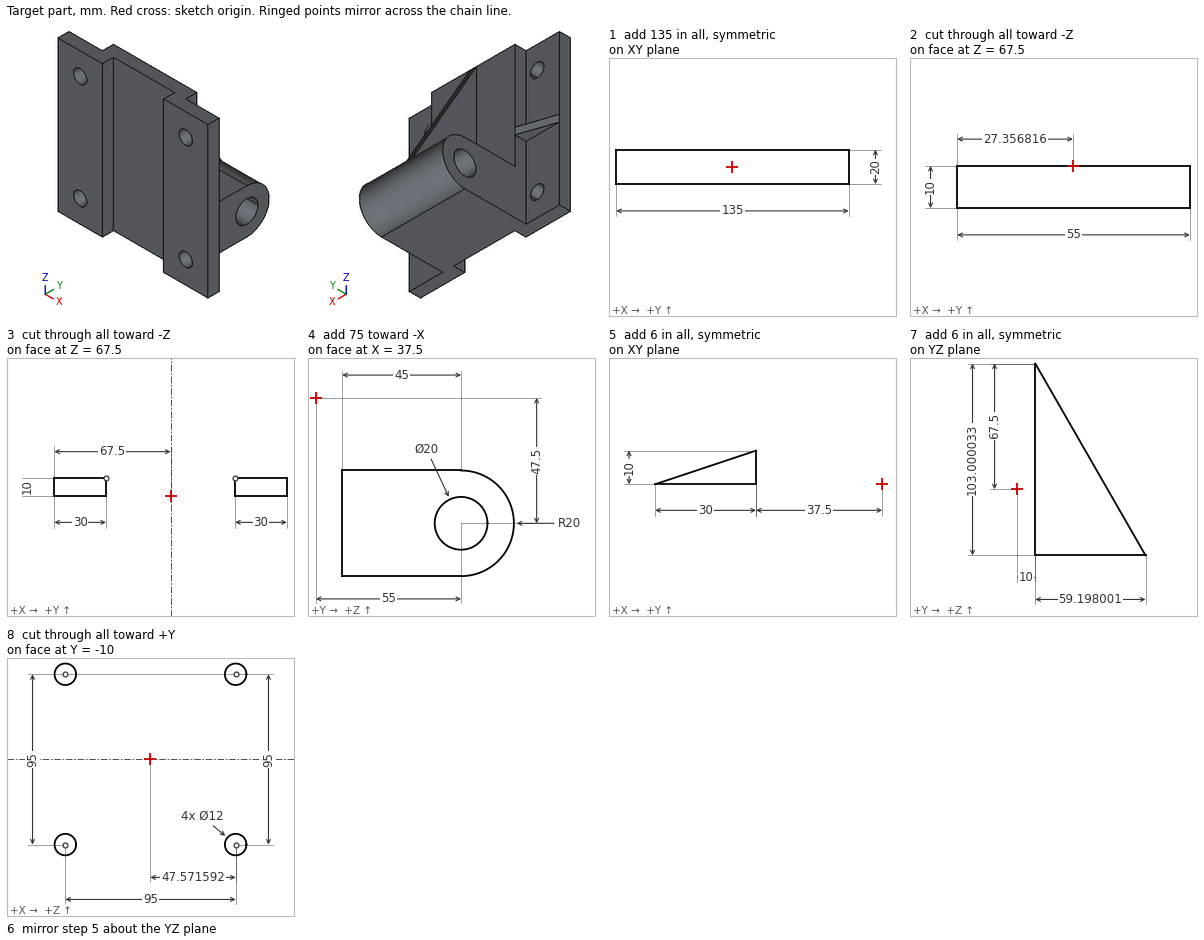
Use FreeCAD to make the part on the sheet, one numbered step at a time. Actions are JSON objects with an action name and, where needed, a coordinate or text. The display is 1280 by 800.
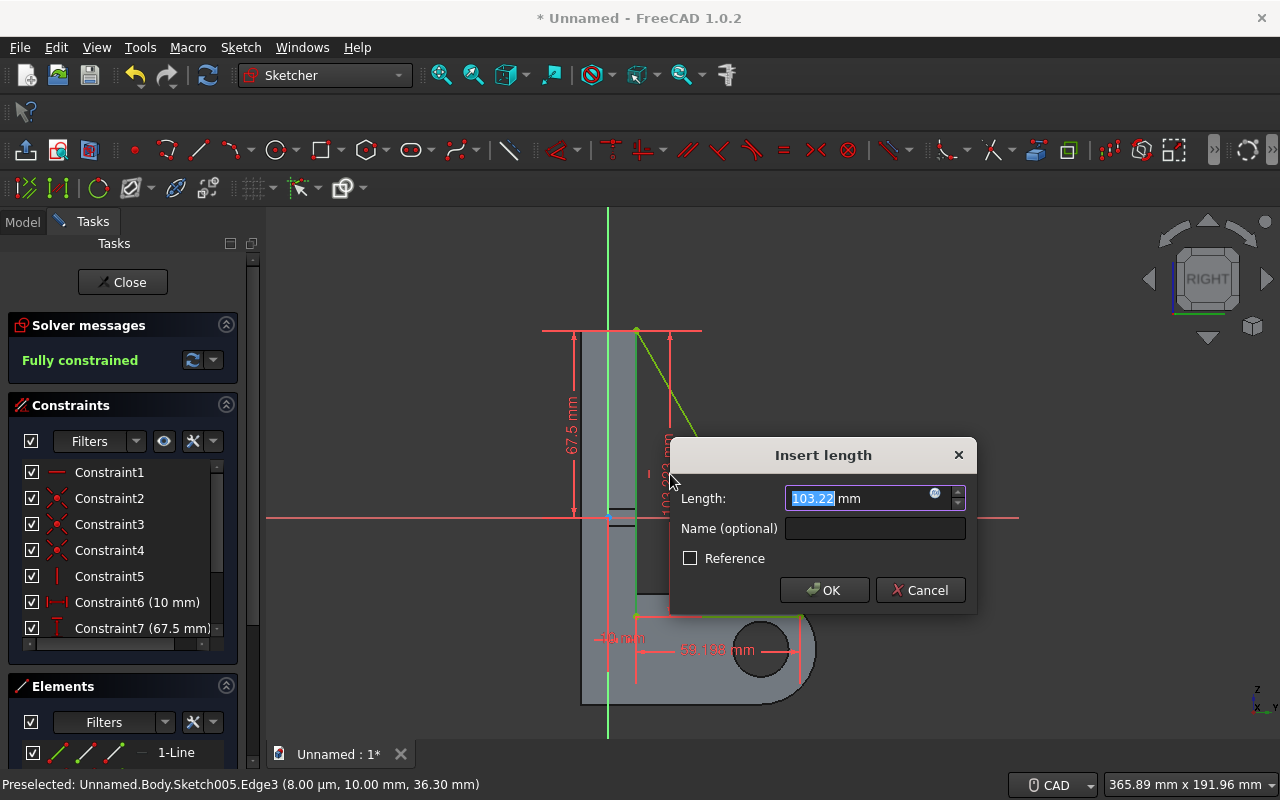
{"action": "type", "text": "103.000033"}
{"action": "key", "text": "Return"}
{"action": "key", "text": "Escape"}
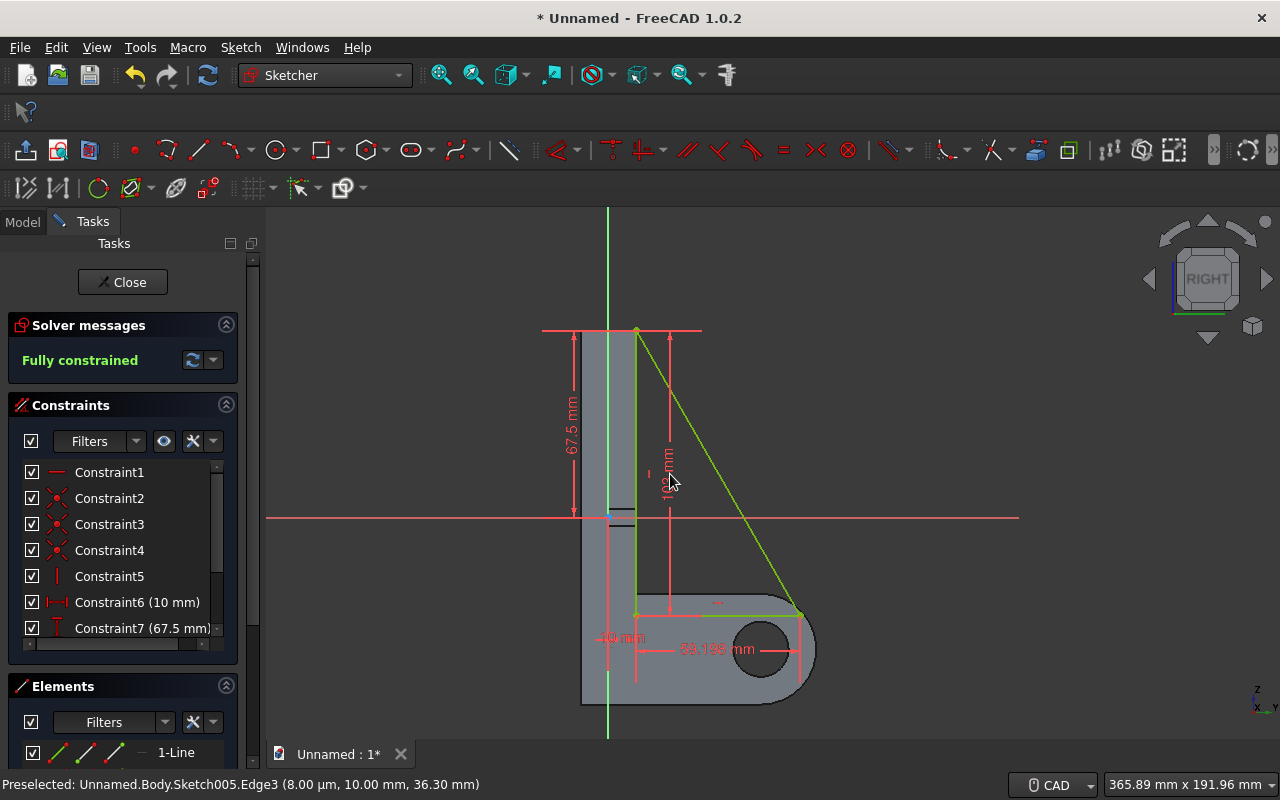
{"action": "left_click", "coordinate": [123, 282]}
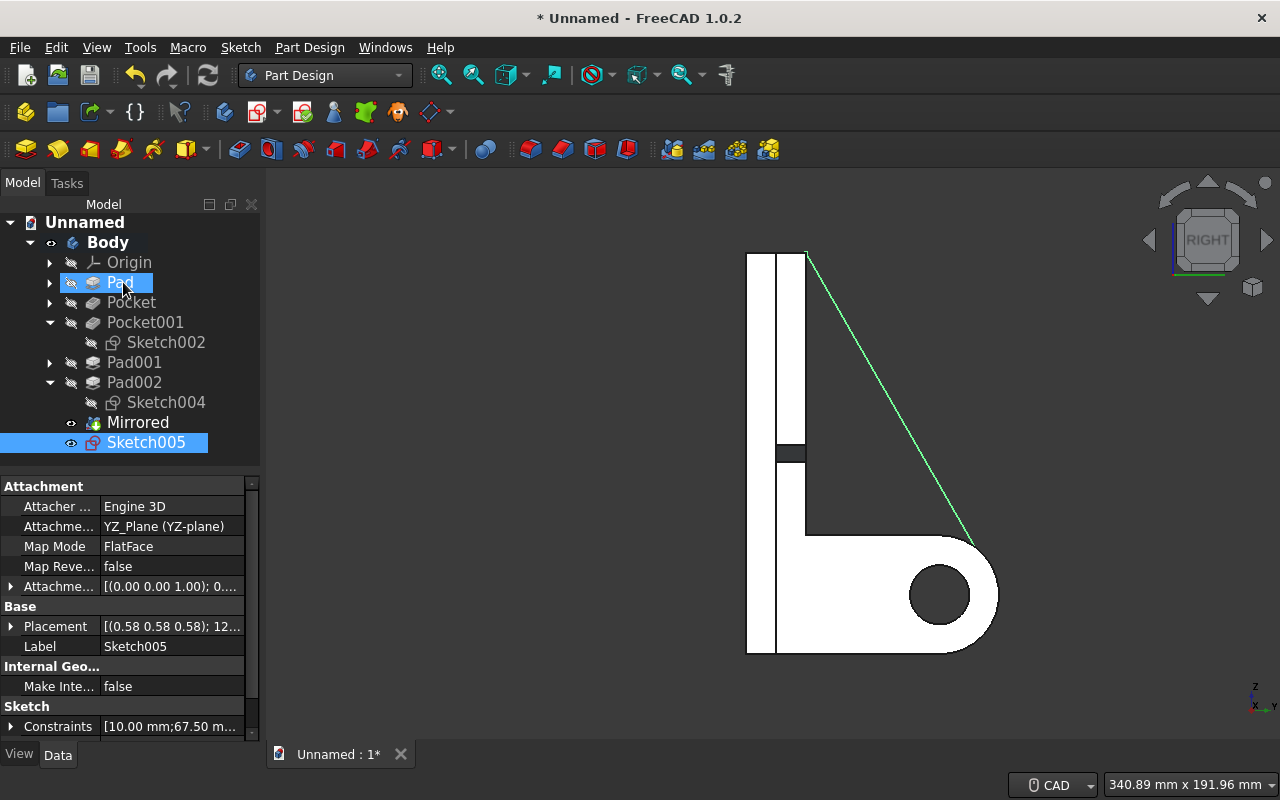
{"action": "left_click", "coordinate": [26, 150]}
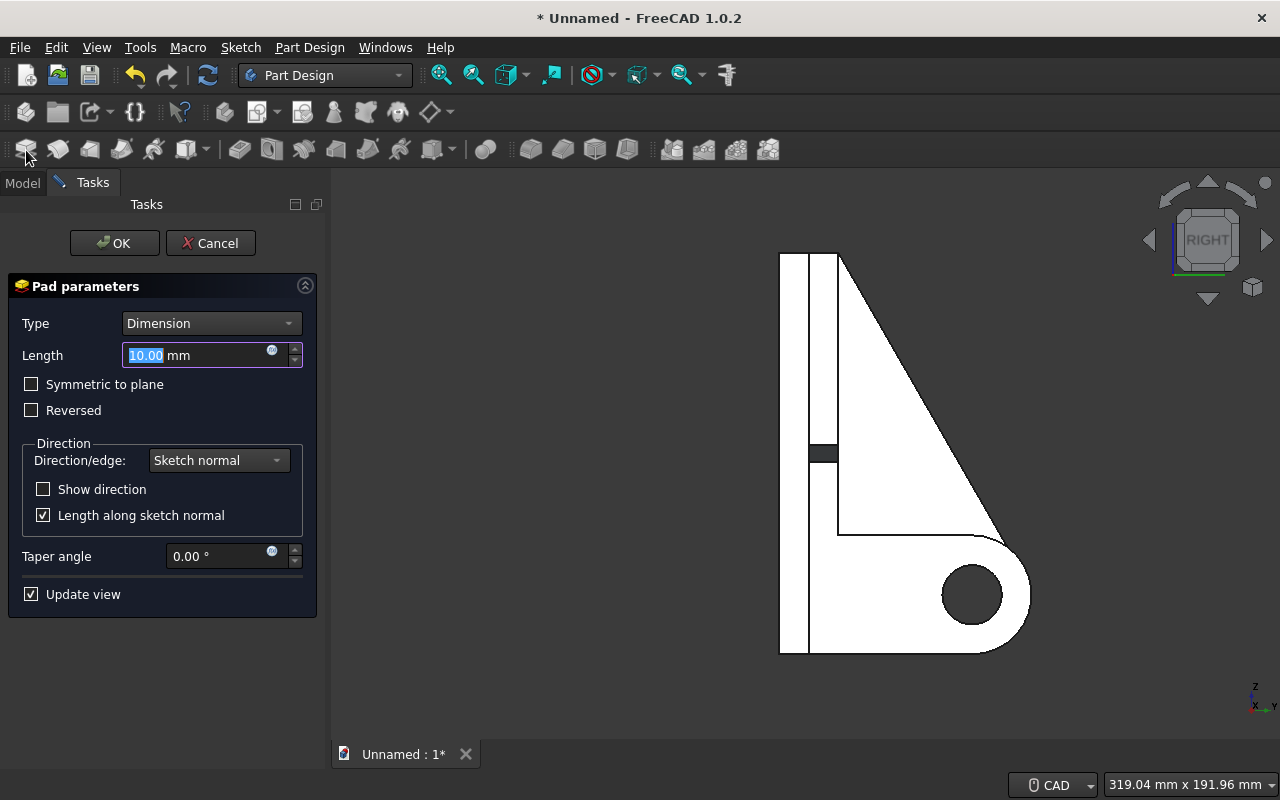
{"action": "type", "text": "6"}
{"action": "key", "text": "Tab"}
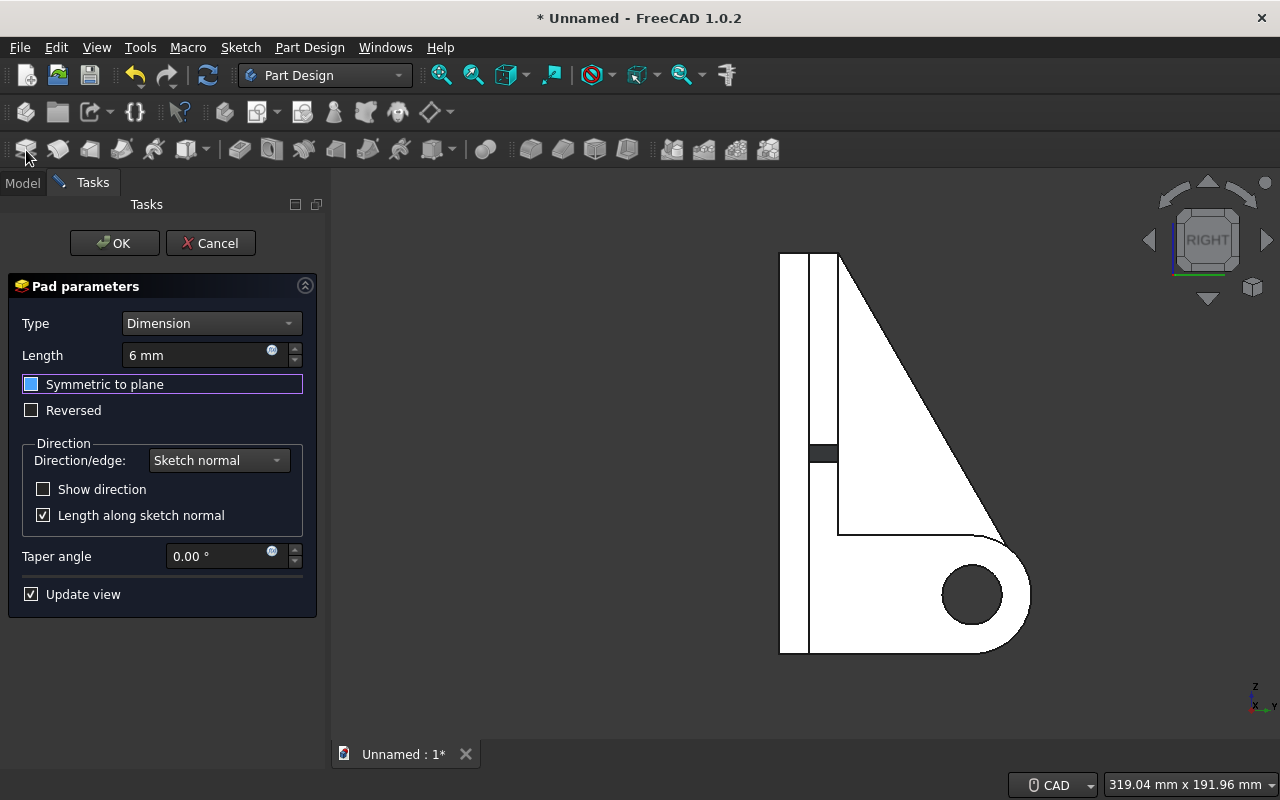
{"action": "left_click", "coordinate": [30, 384]}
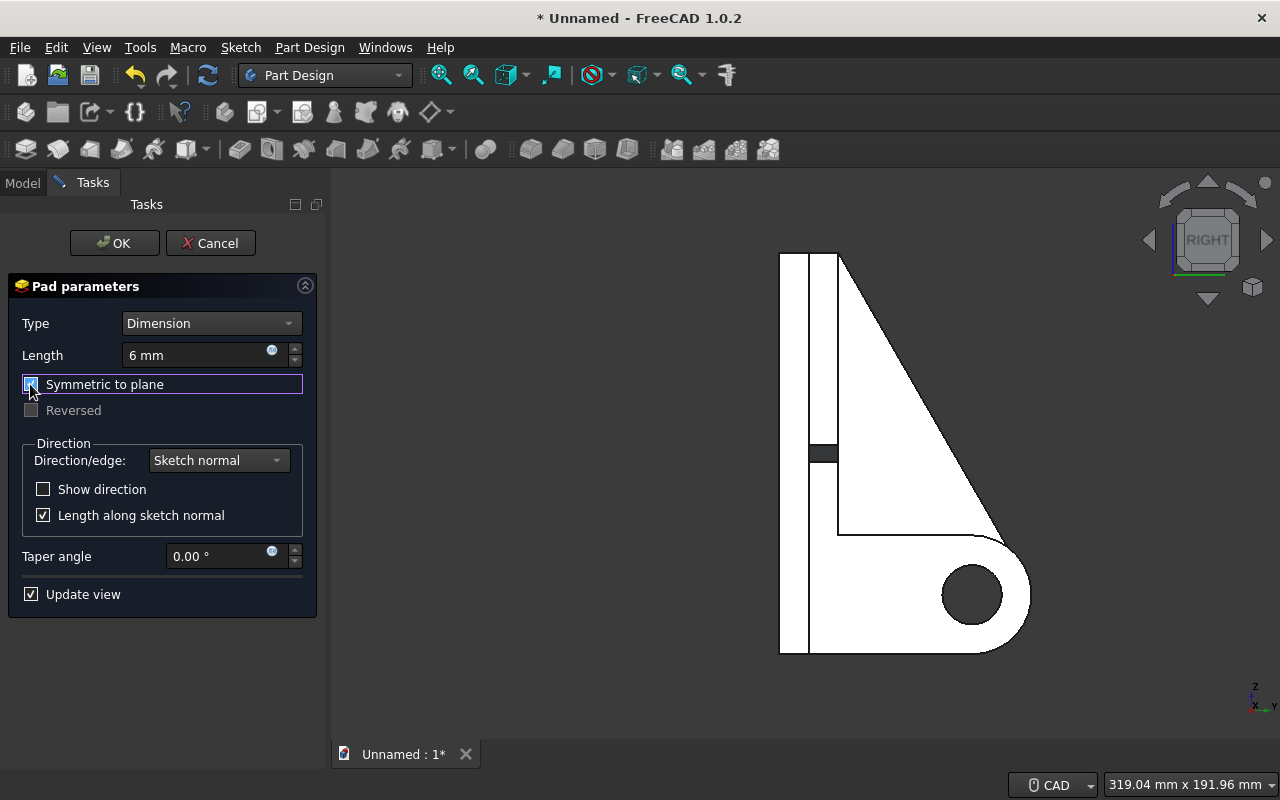
{"action": "left_click", "coordinate": [115, 243]}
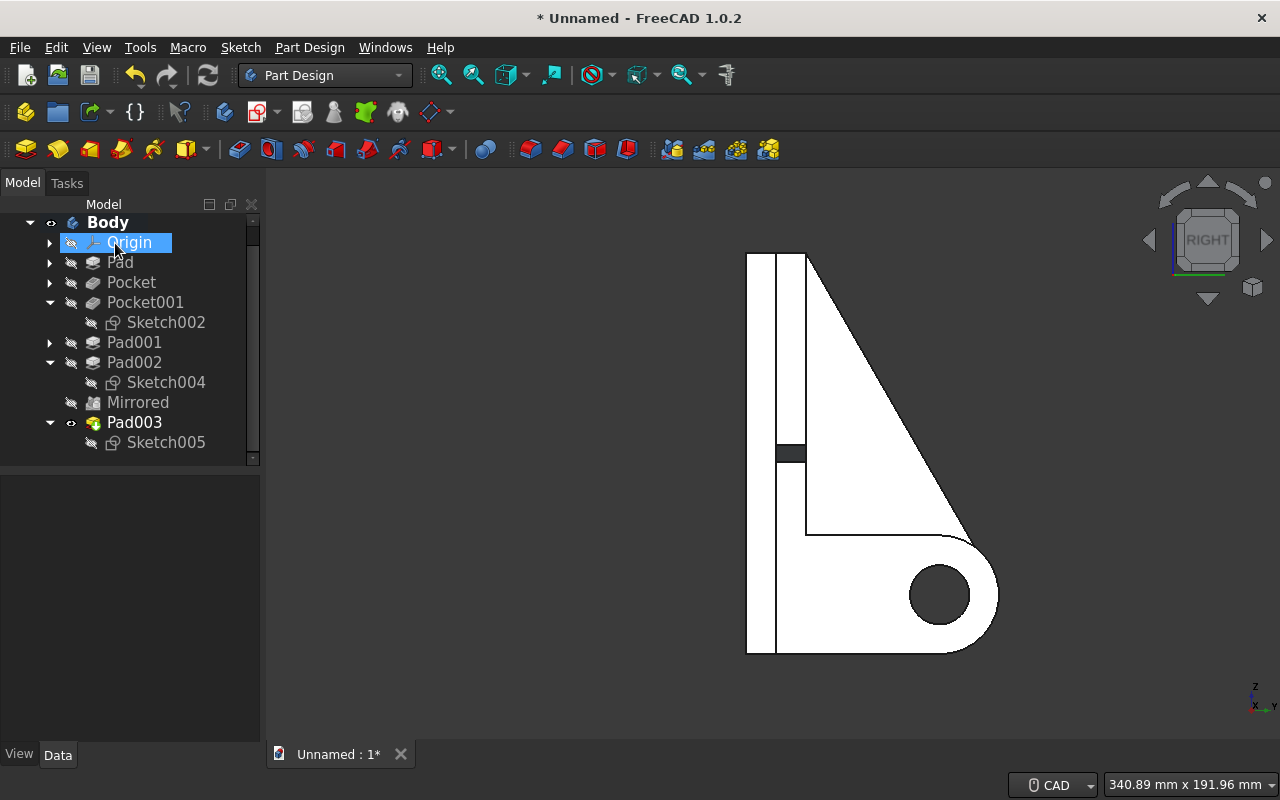
{"action": "key", "text": "0"}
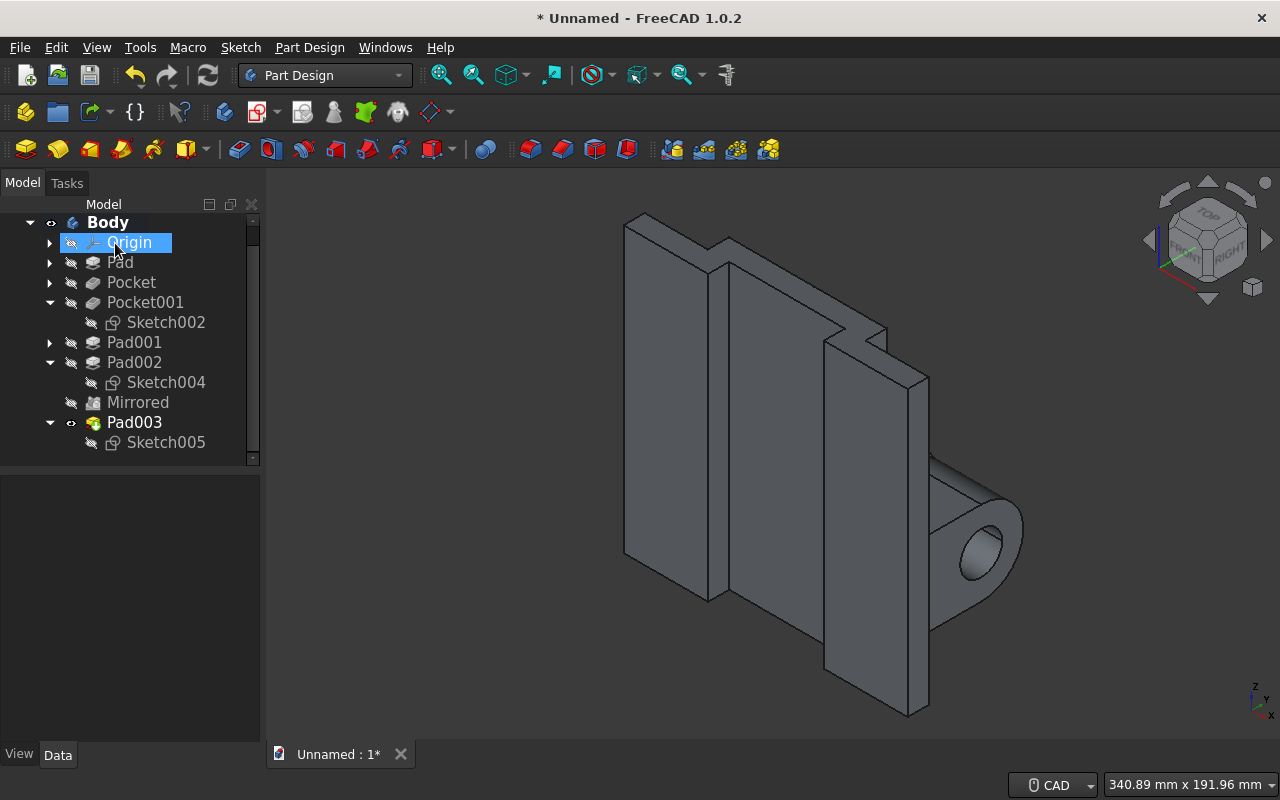
{"action": "left_click", "coordinate": [442, 76]}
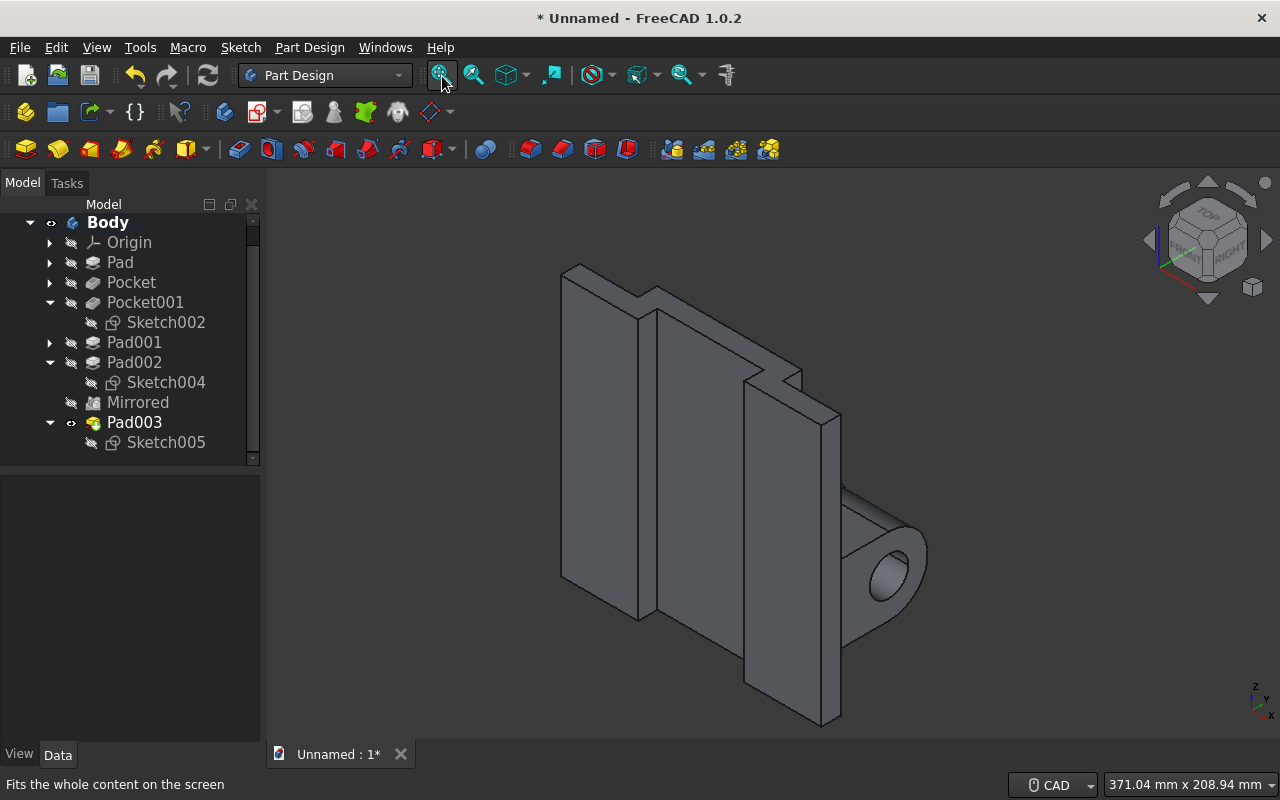
{"action": "left_click", "coordinate": [599, 361]}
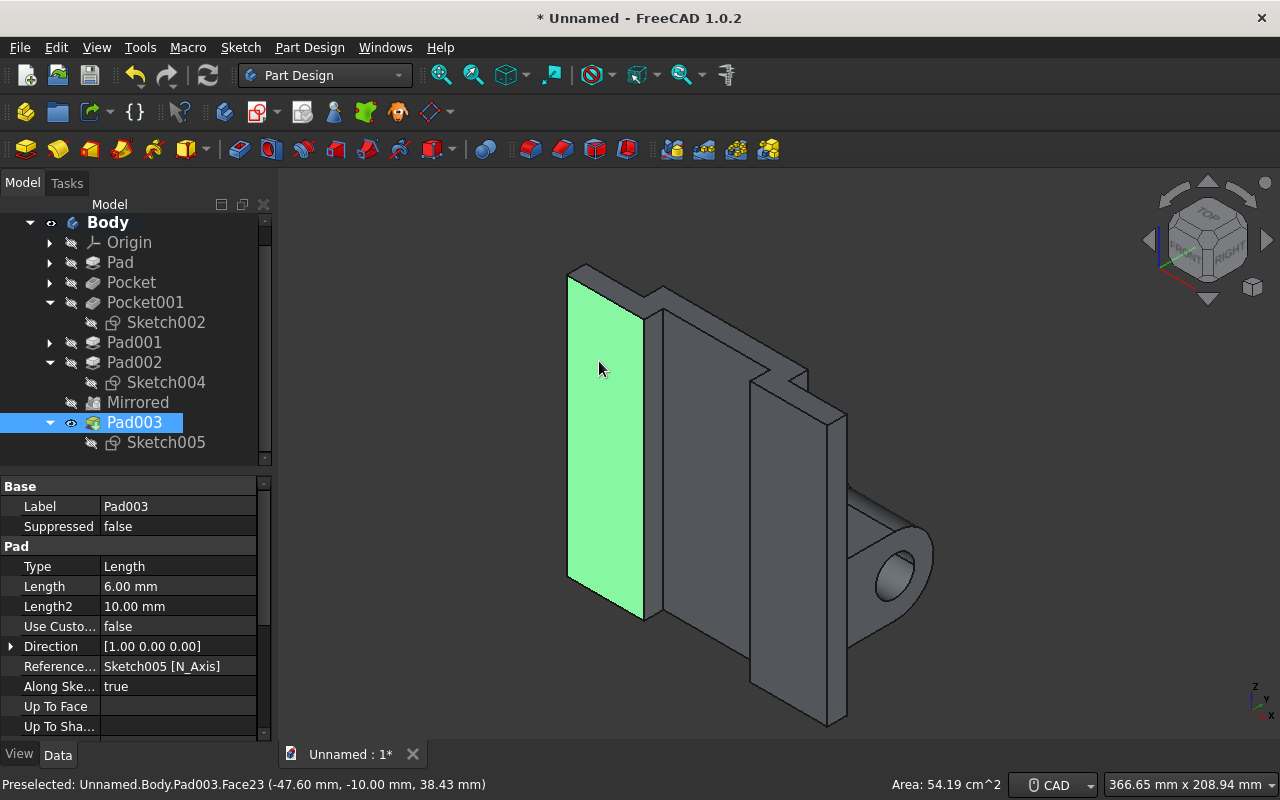
{"action": "left_click", "coordinate": [258, 112]}